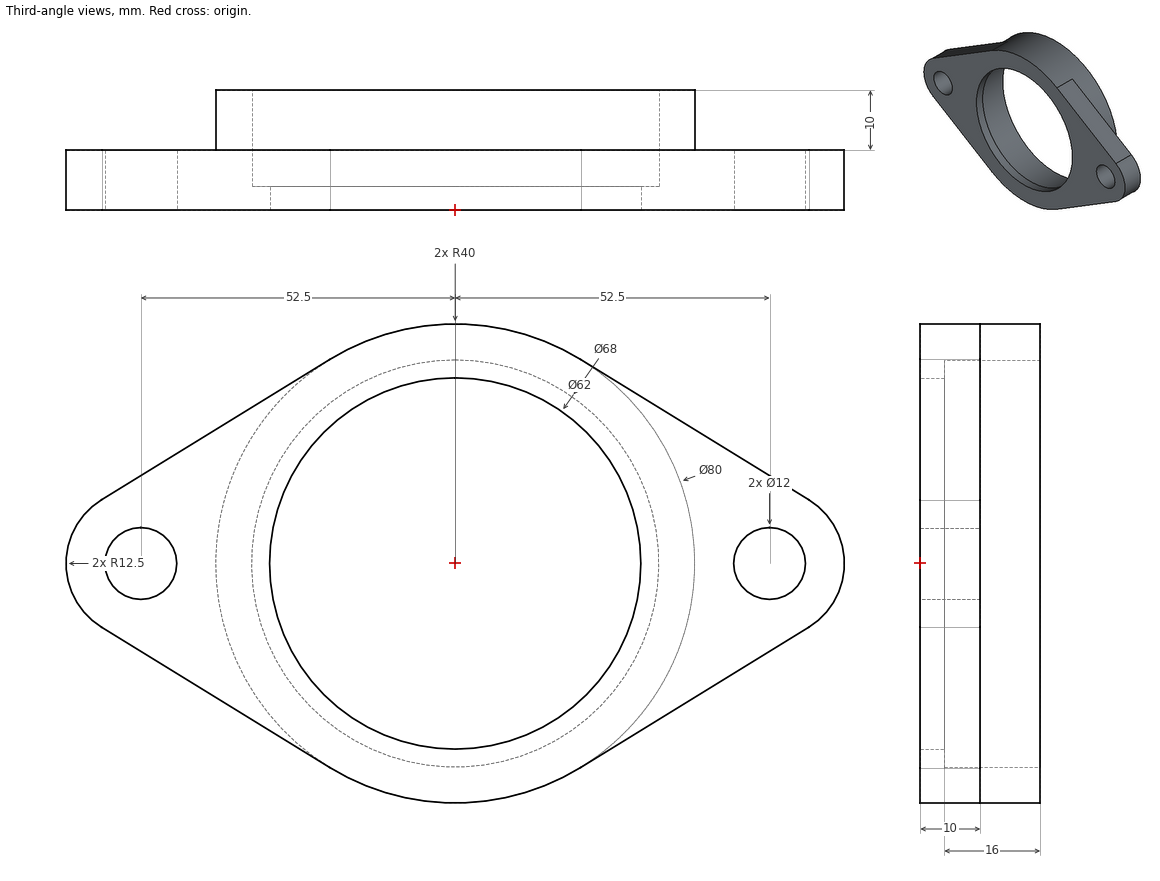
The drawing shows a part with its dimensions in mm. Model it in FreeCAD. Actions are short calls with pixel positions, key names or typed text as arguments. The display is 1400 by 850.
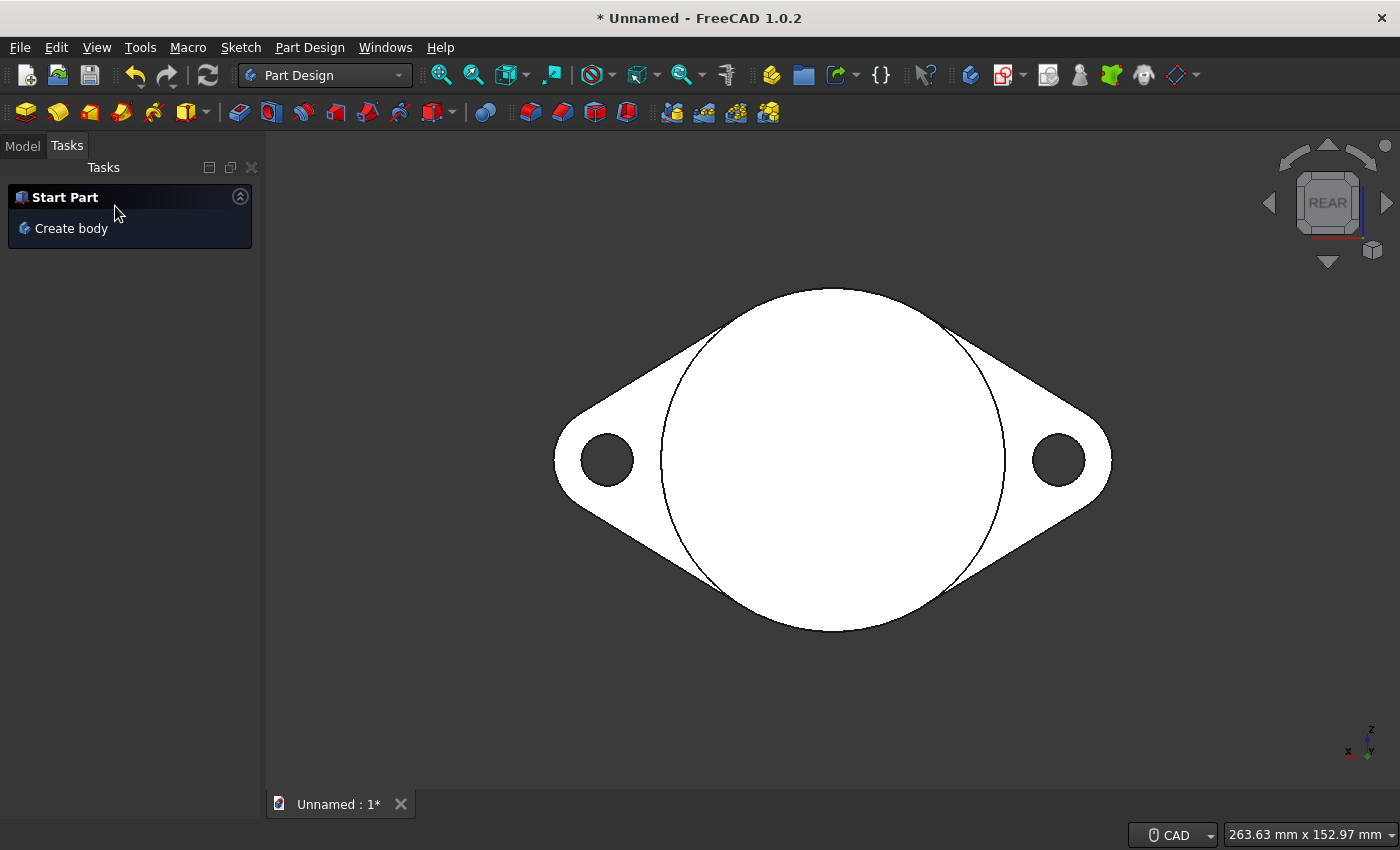
click(833, 459)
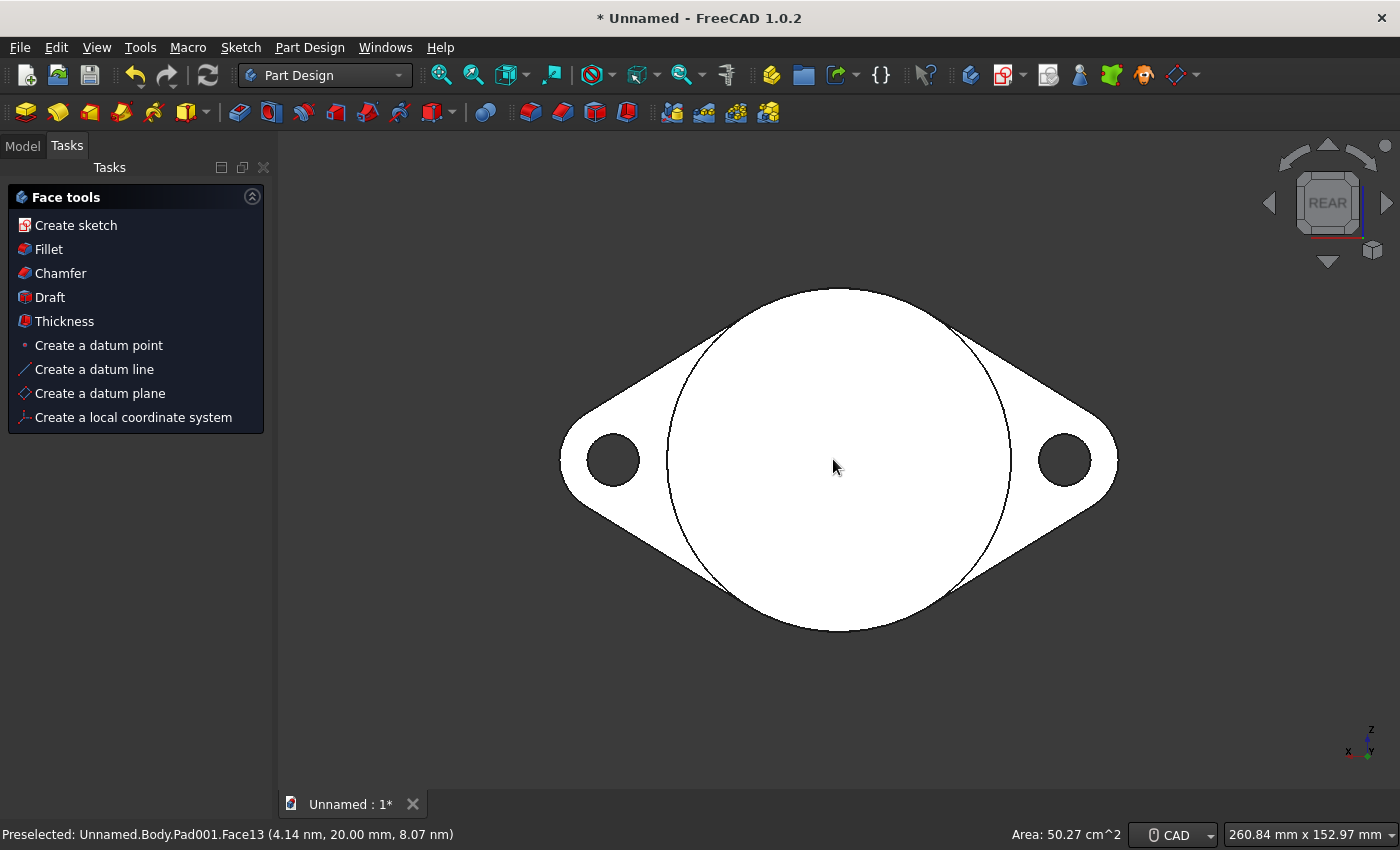
click(1004, 76)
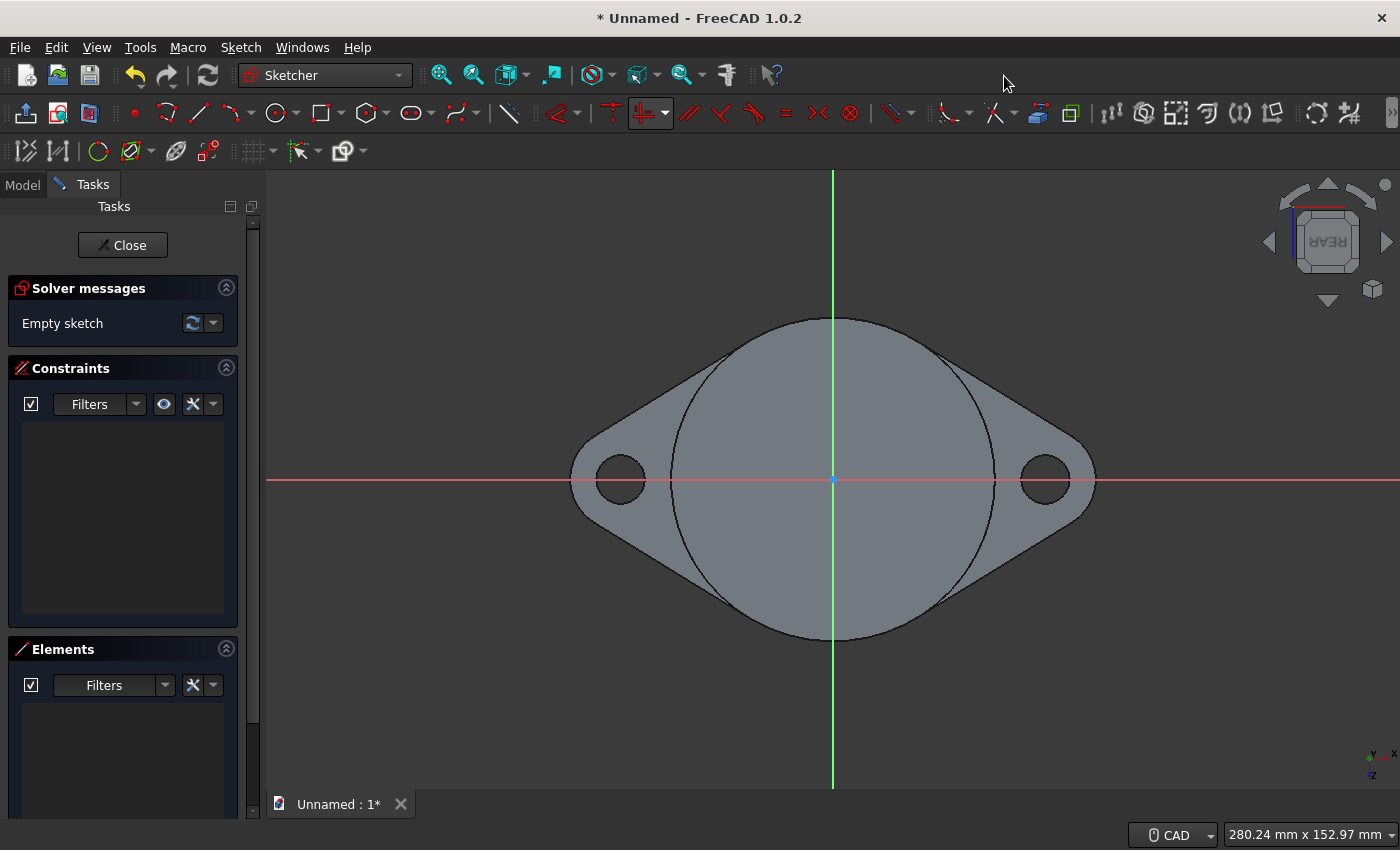
scroll(972, 479, up, 2)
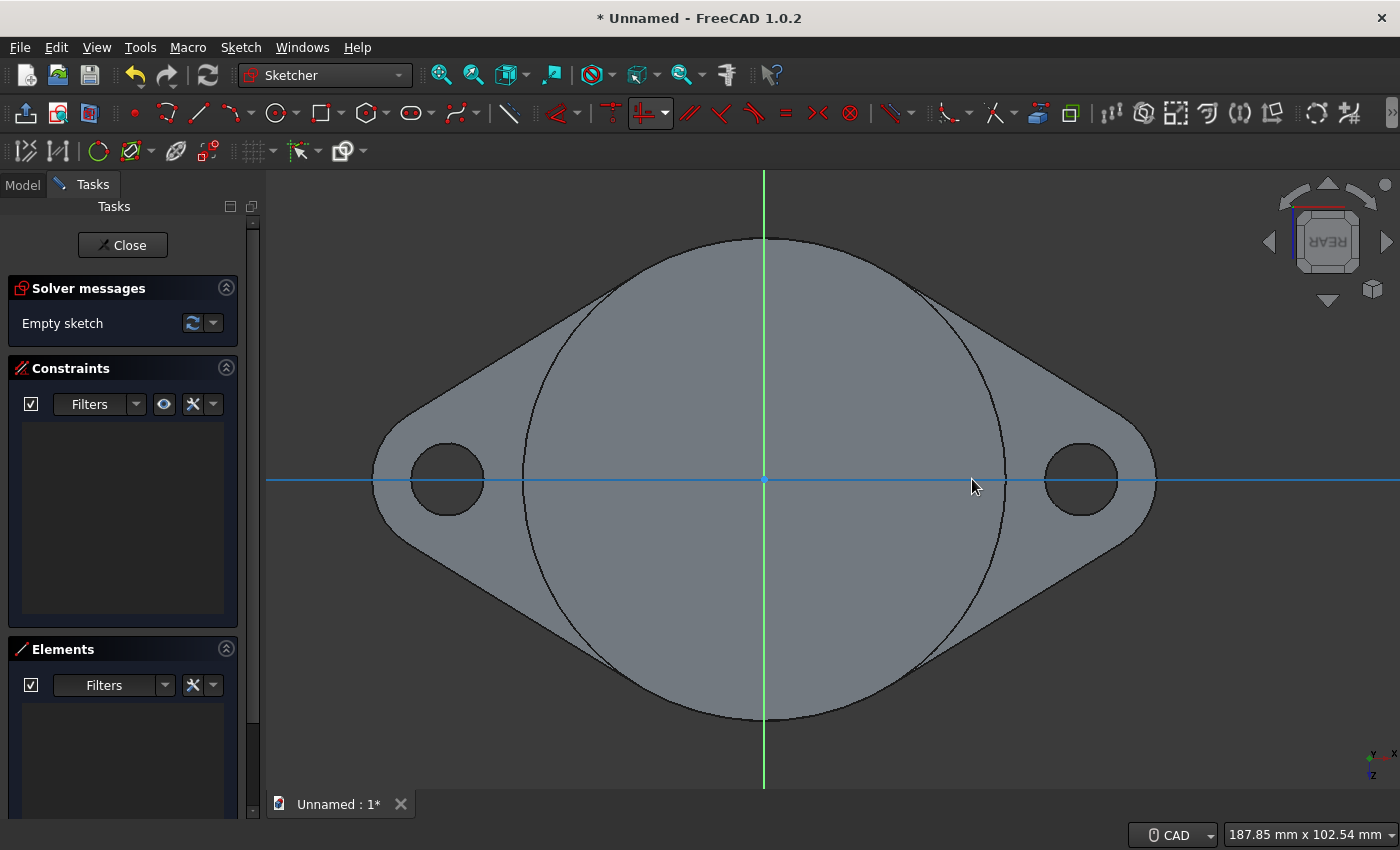
click(276, 114)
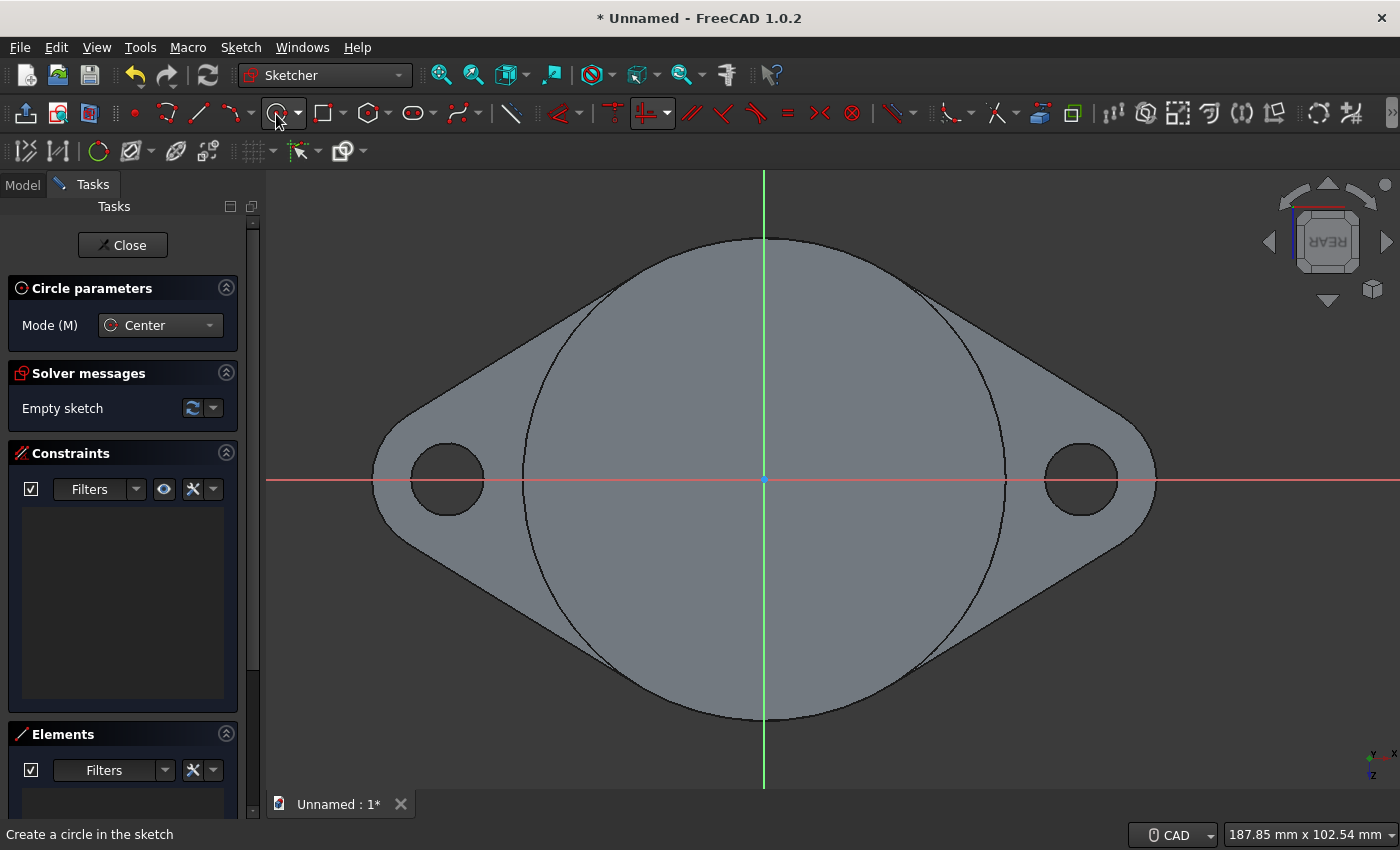
click(764, 479)
move(909, 334)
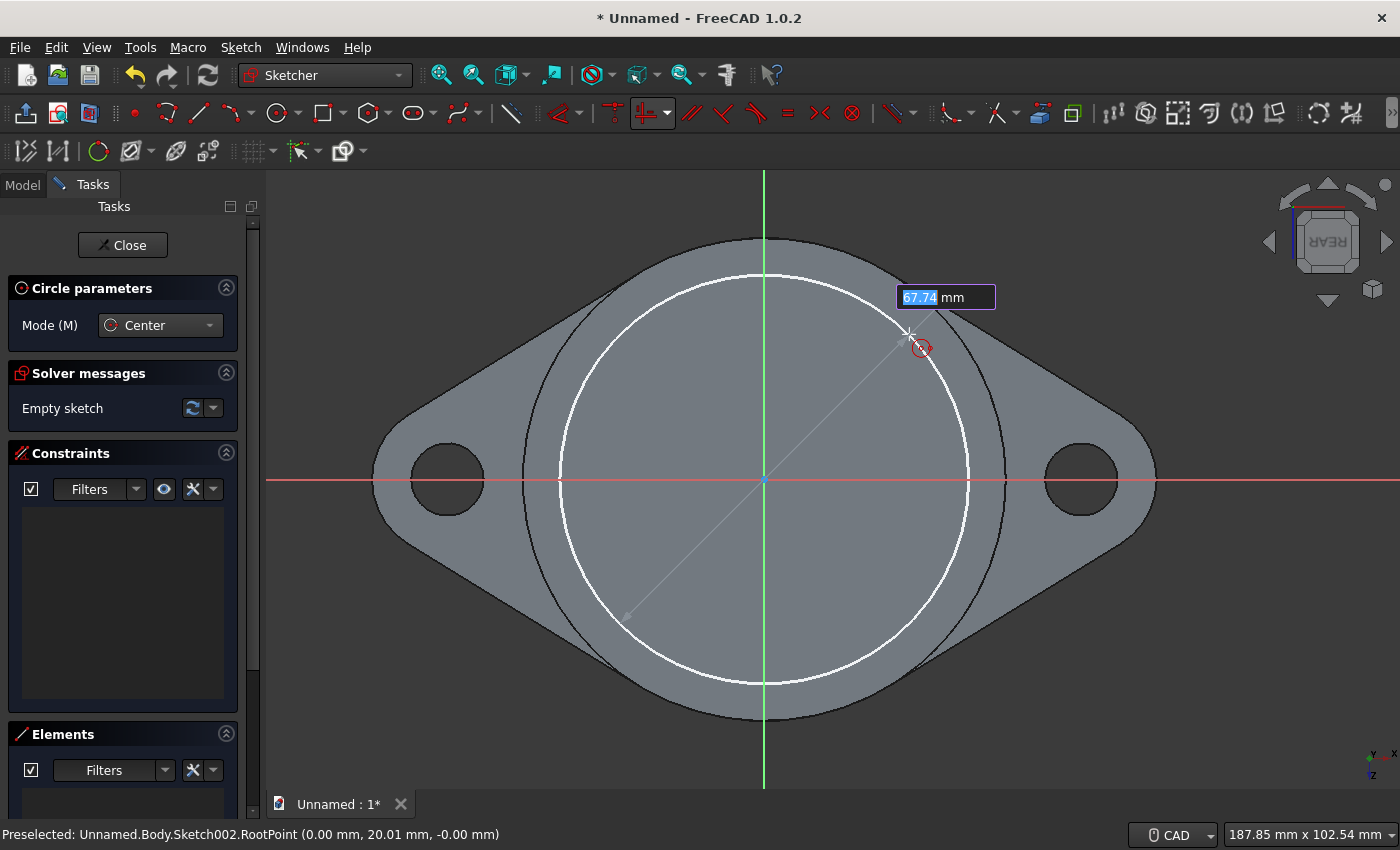
text(68)
key(Return)
key(Escape)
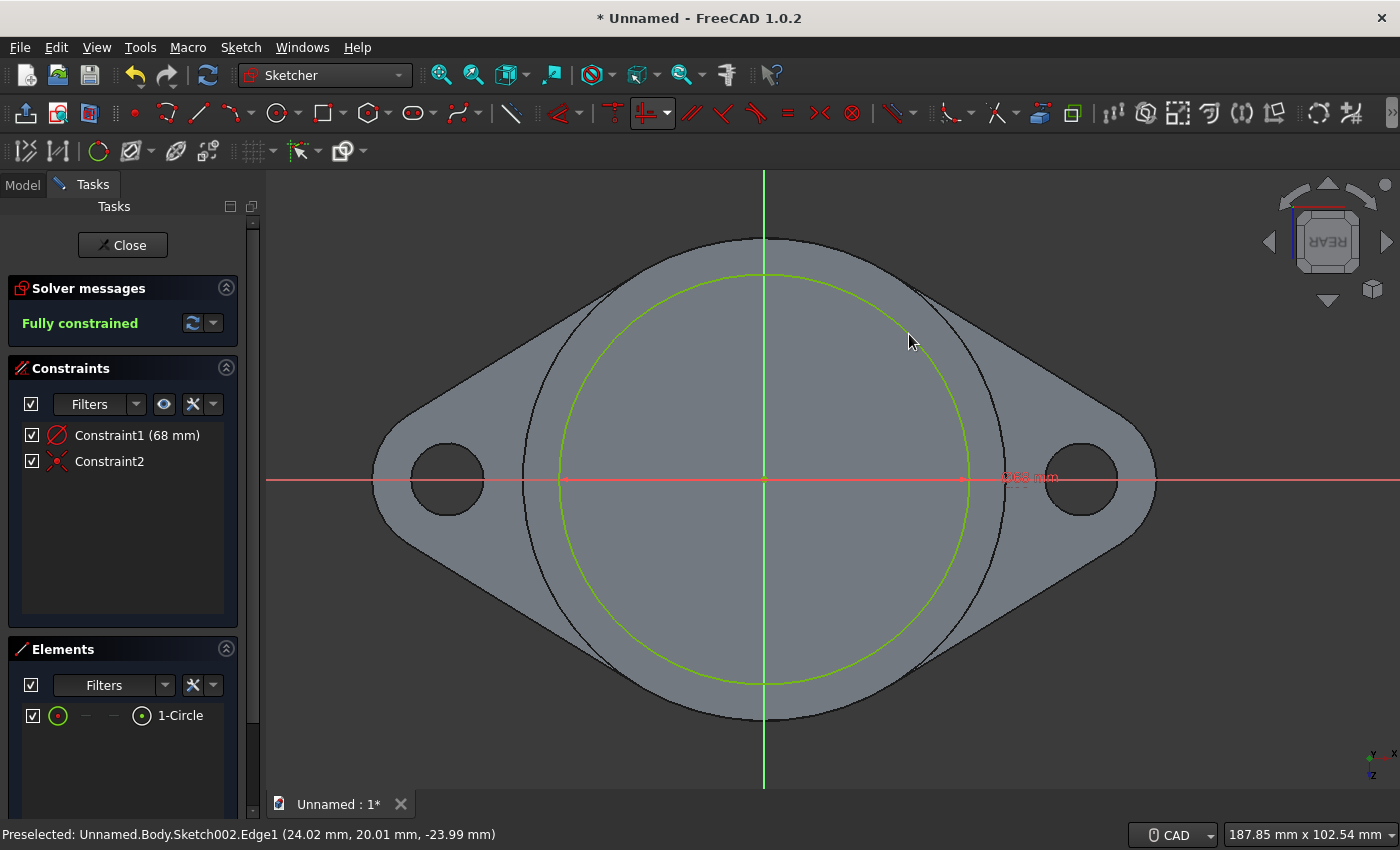
click(123, 245)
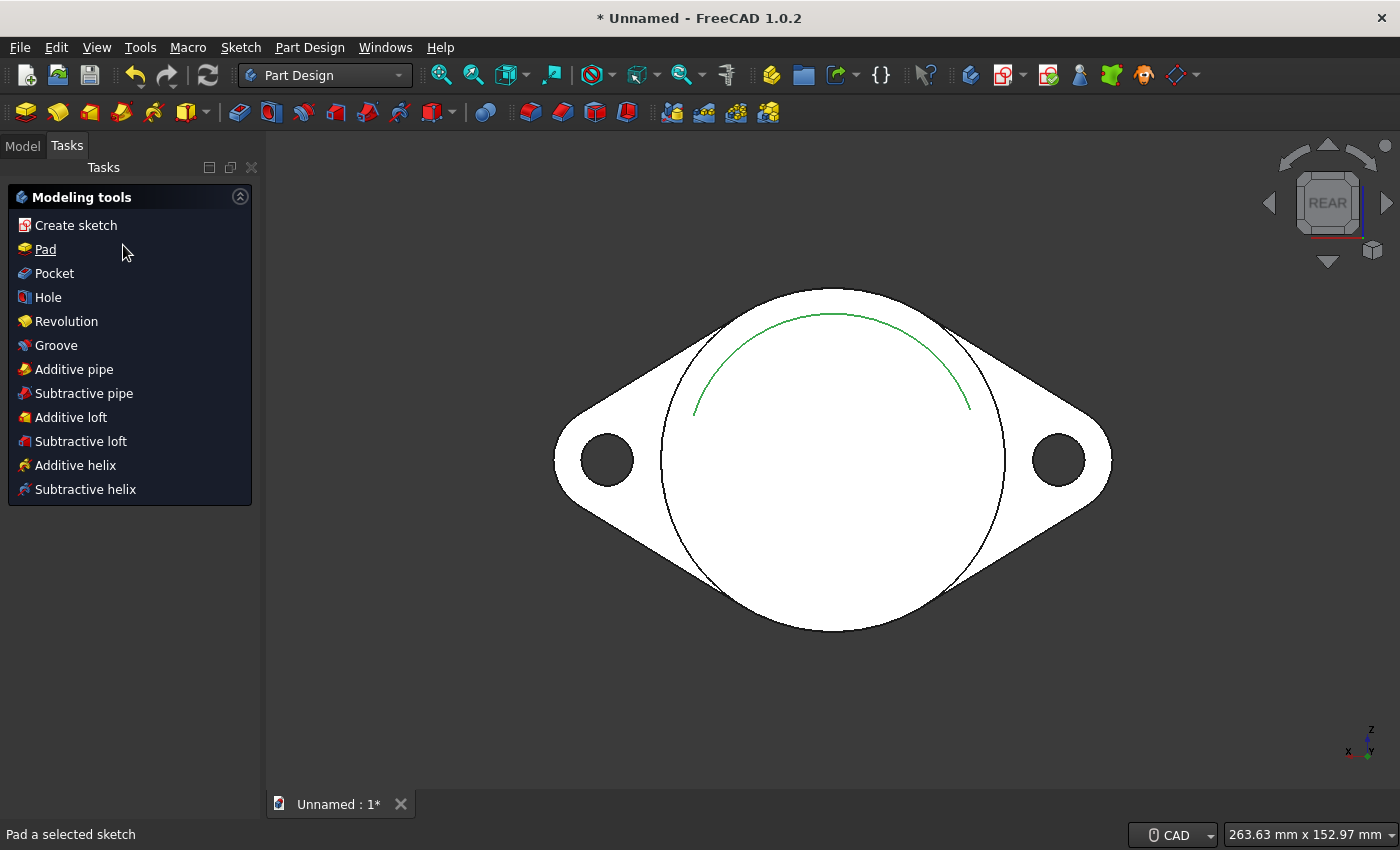
click(240, 112)